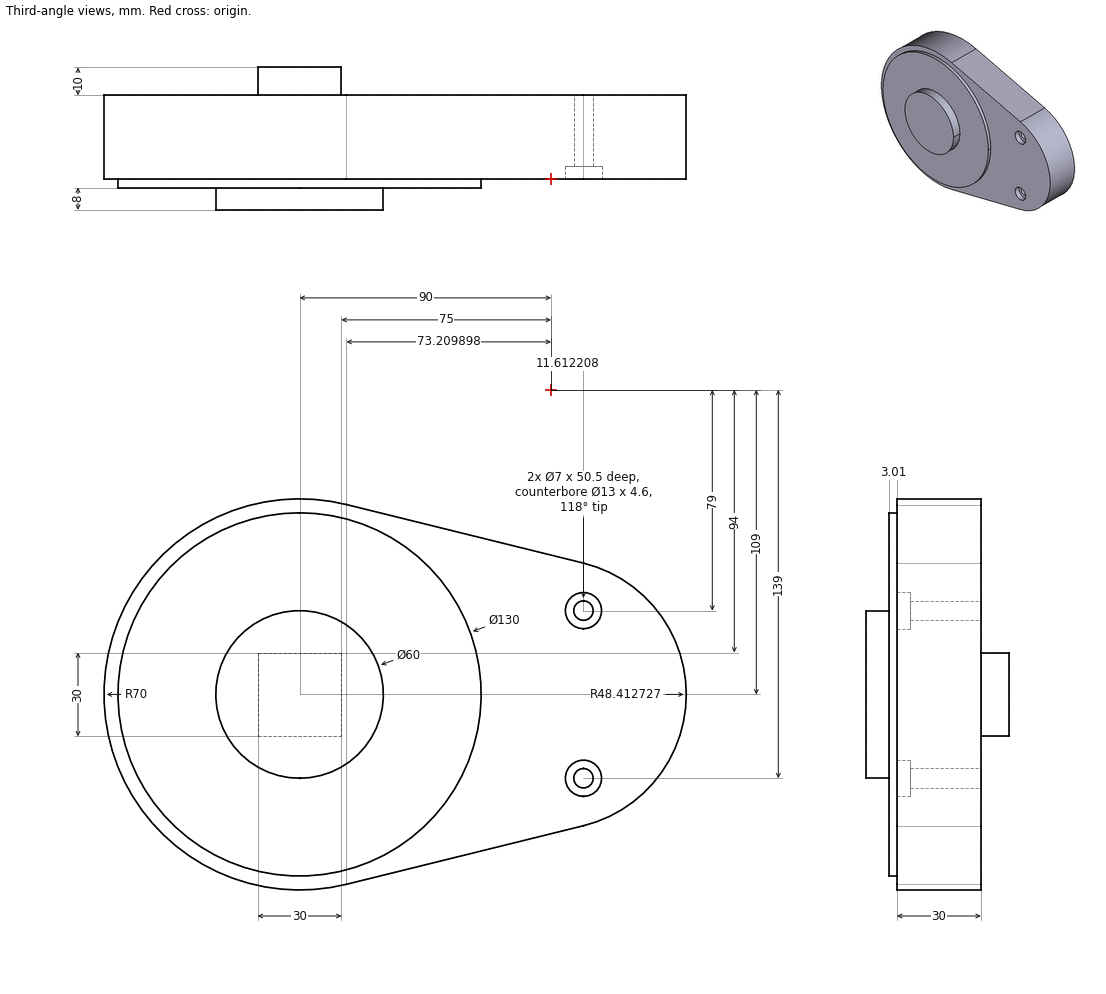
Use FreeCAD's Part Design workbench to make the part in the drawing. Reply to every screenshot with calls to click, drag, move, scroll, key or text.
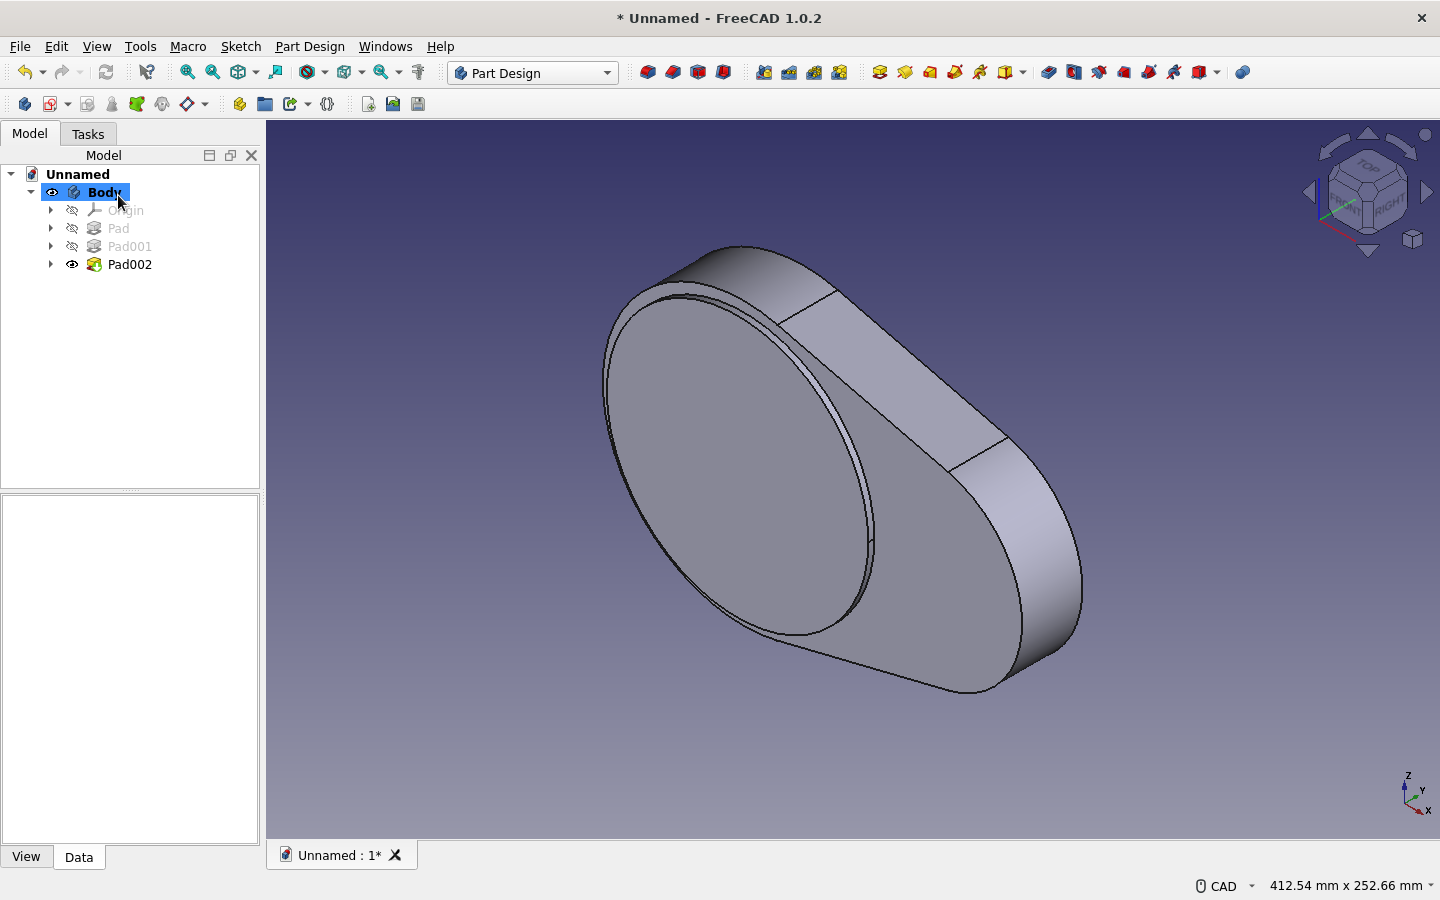
click(738, 466)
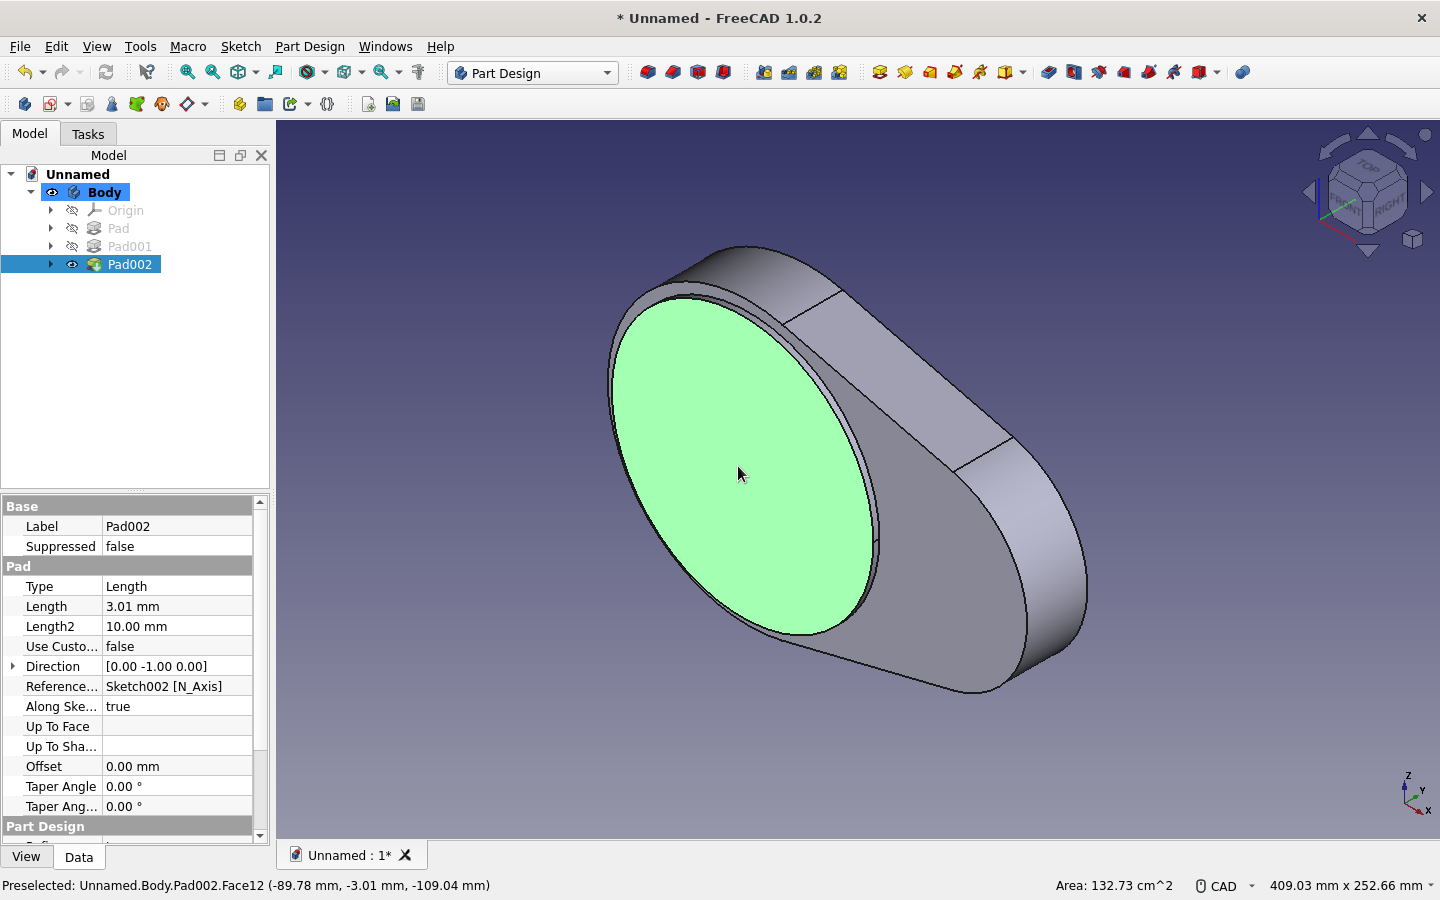
click(50, 104)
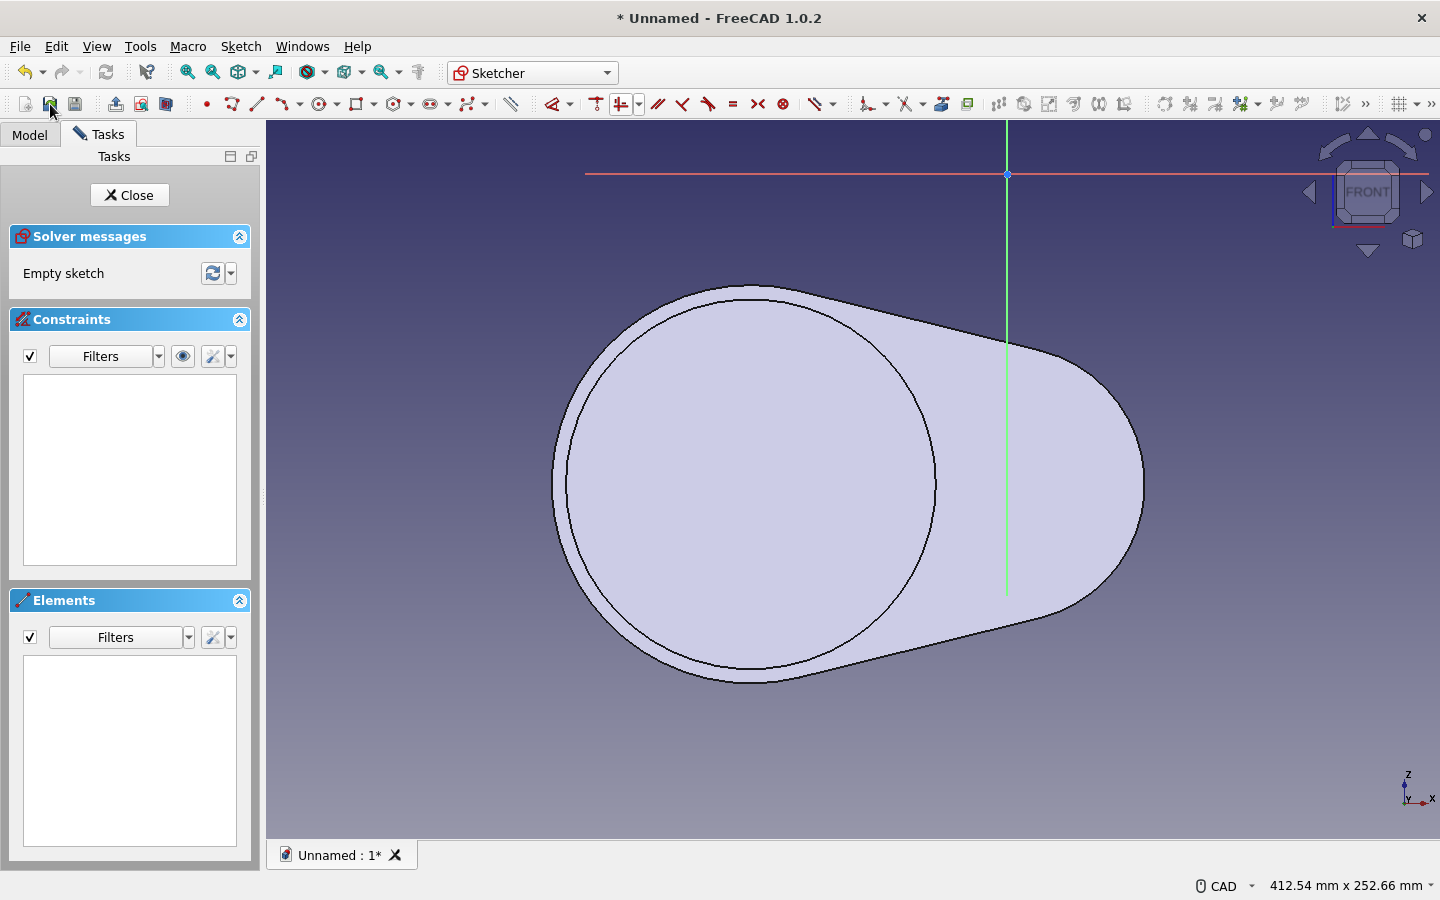
key(g)
key(c)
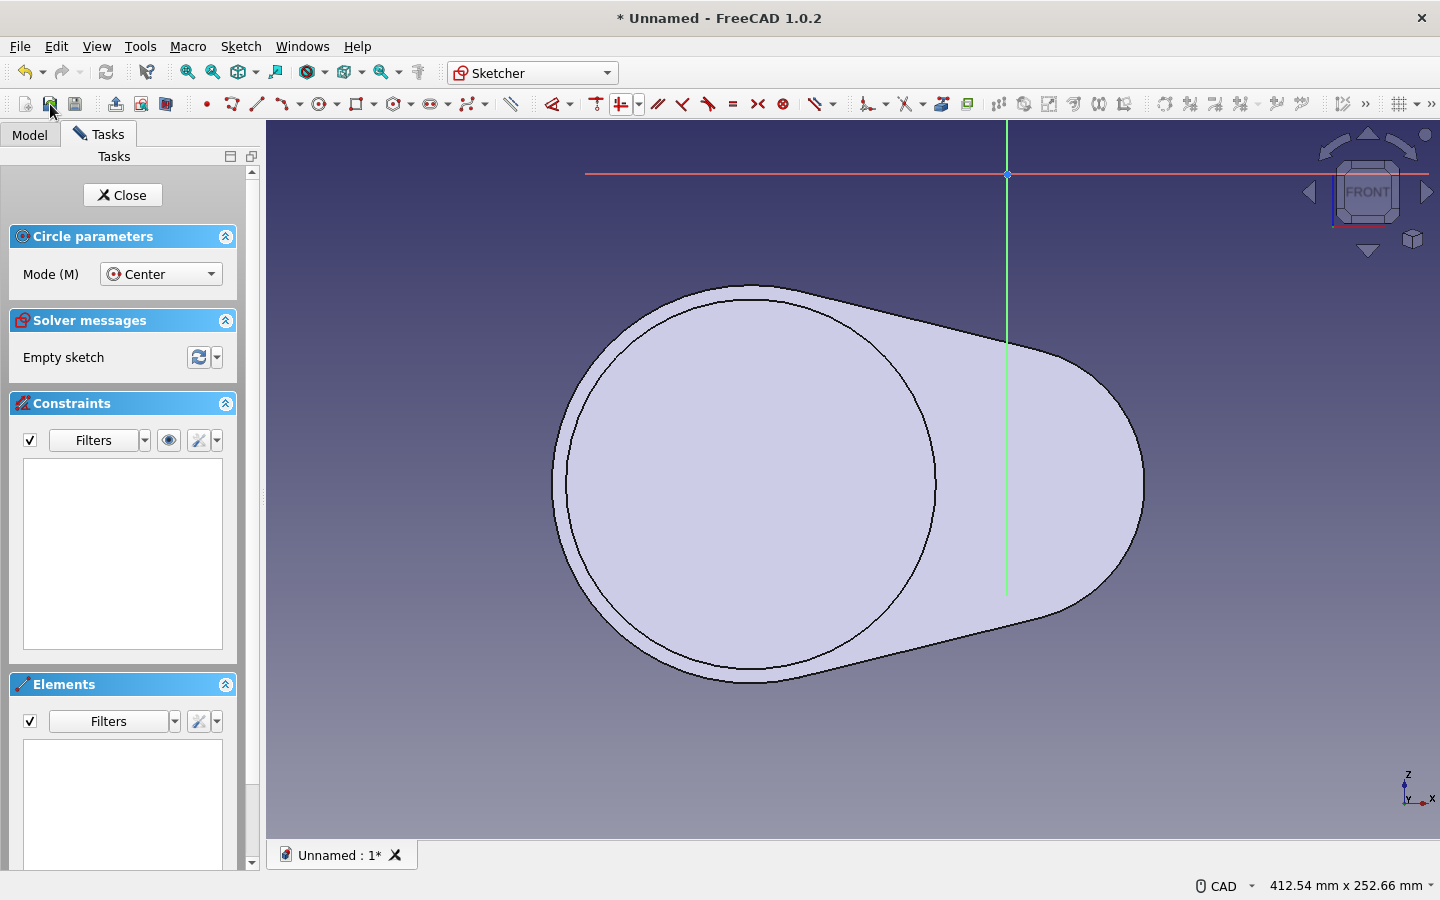
click(751, 484)
click(811, 424)
key(Escape)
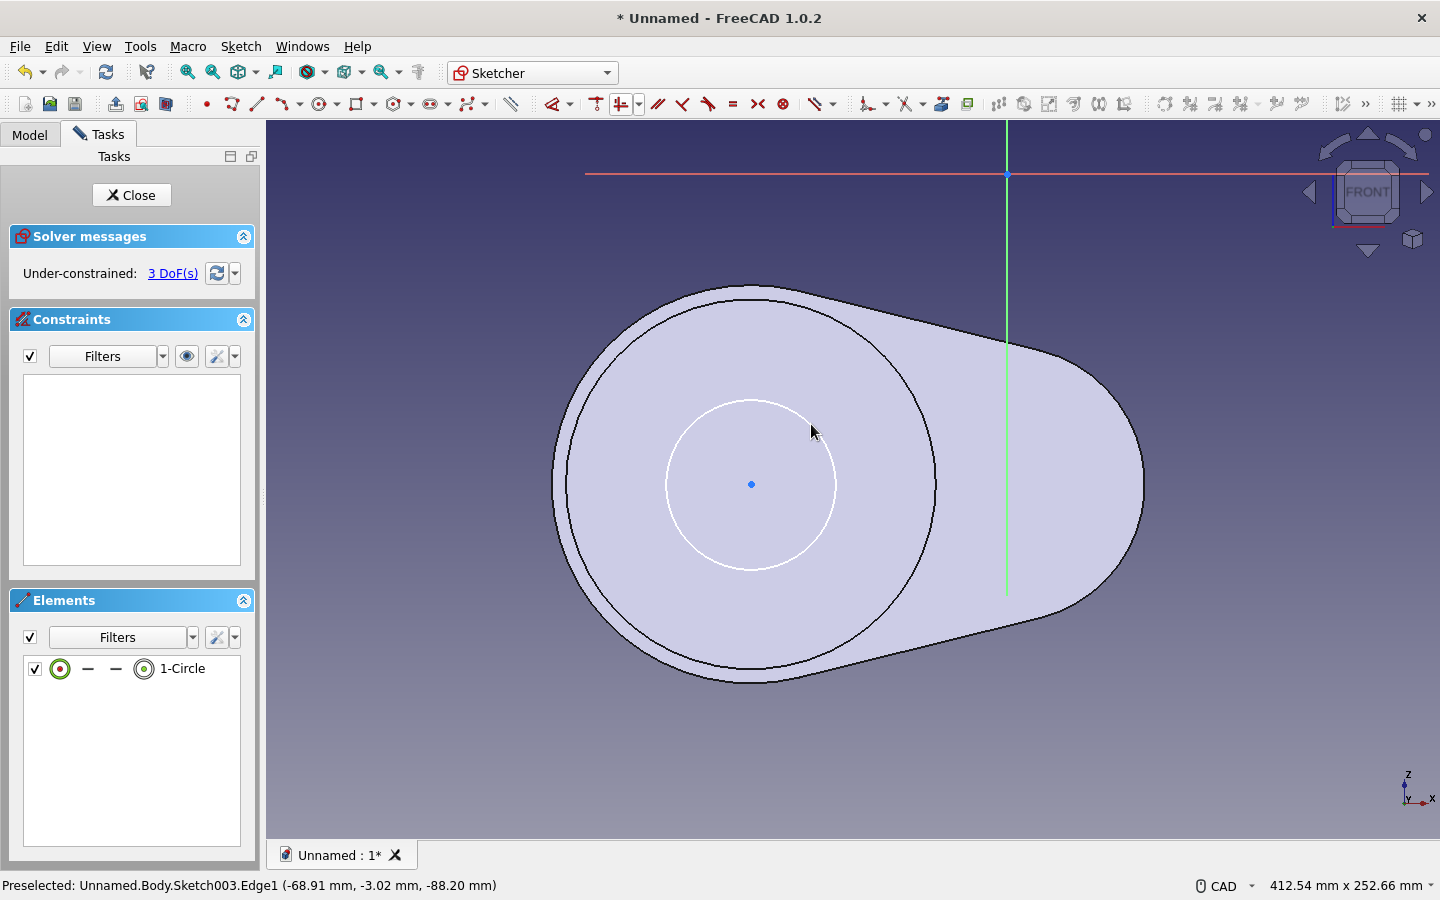
click(552, 104)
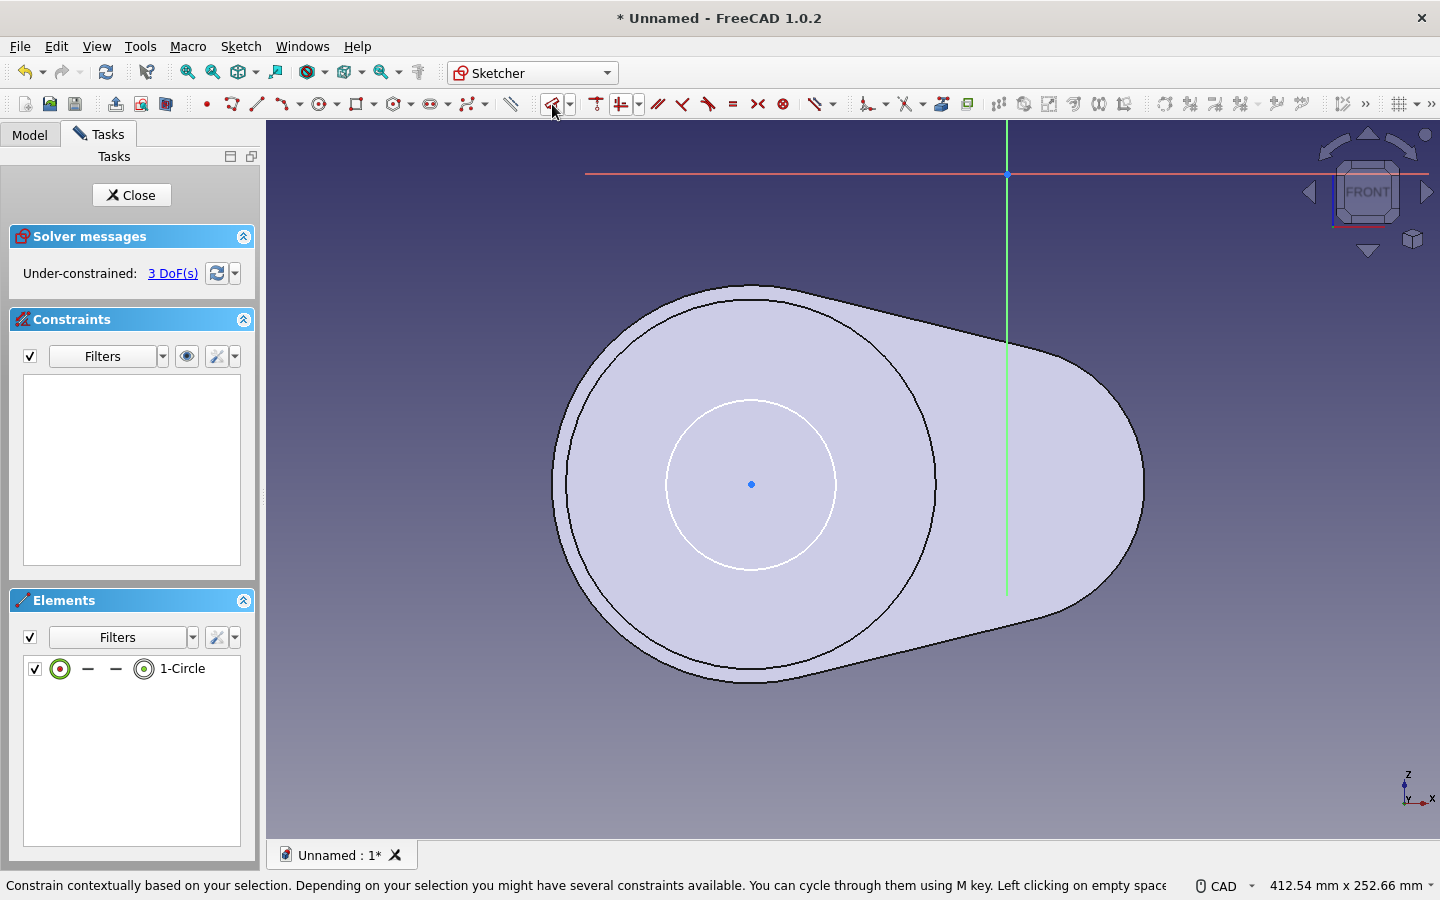
click(811, 425)
click(834, 402)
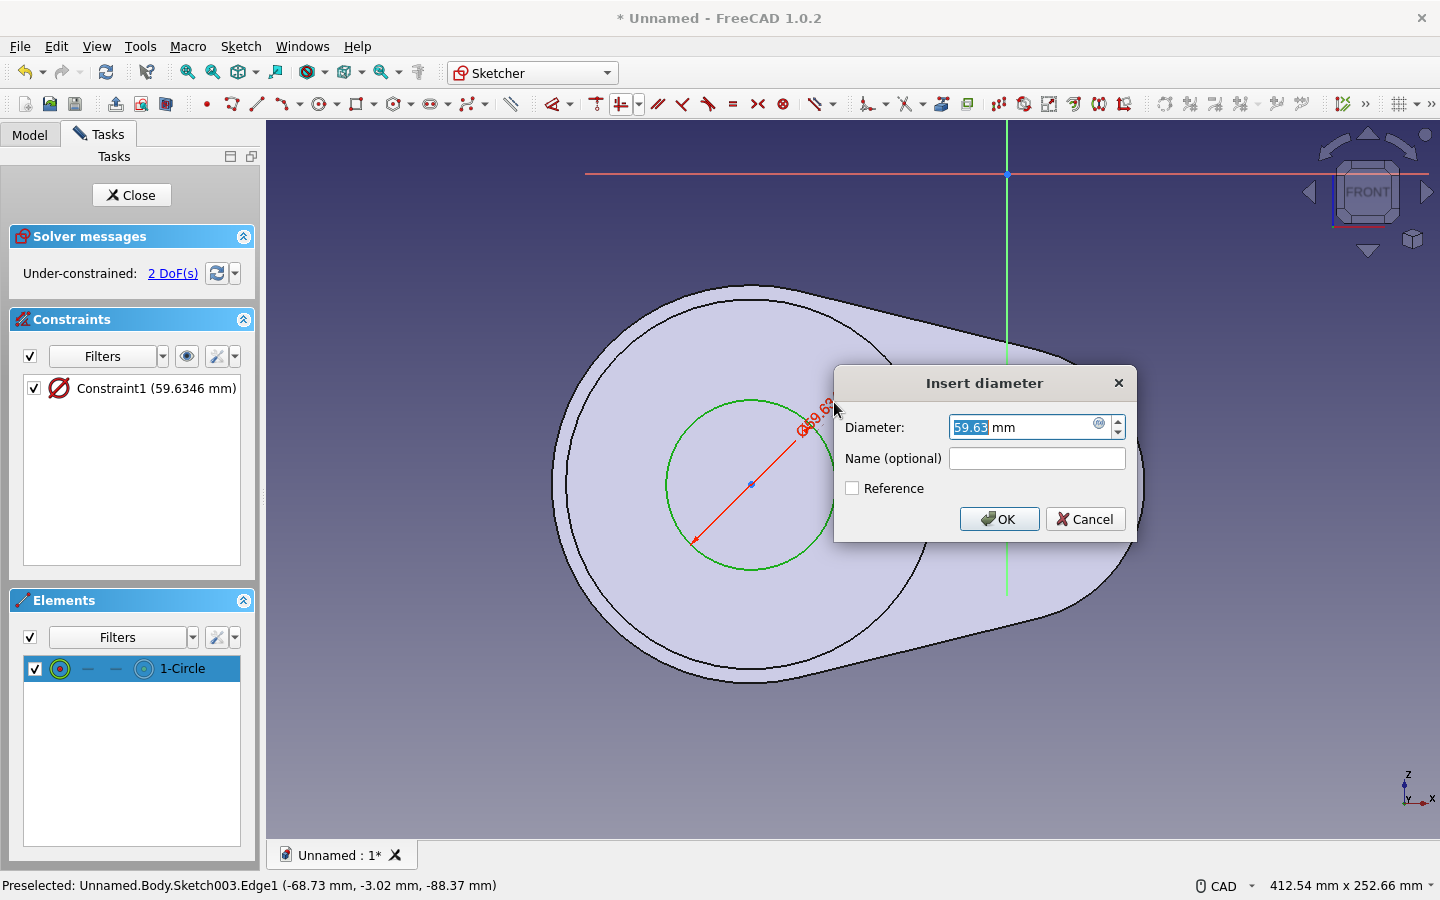
text(60)
key(Return)